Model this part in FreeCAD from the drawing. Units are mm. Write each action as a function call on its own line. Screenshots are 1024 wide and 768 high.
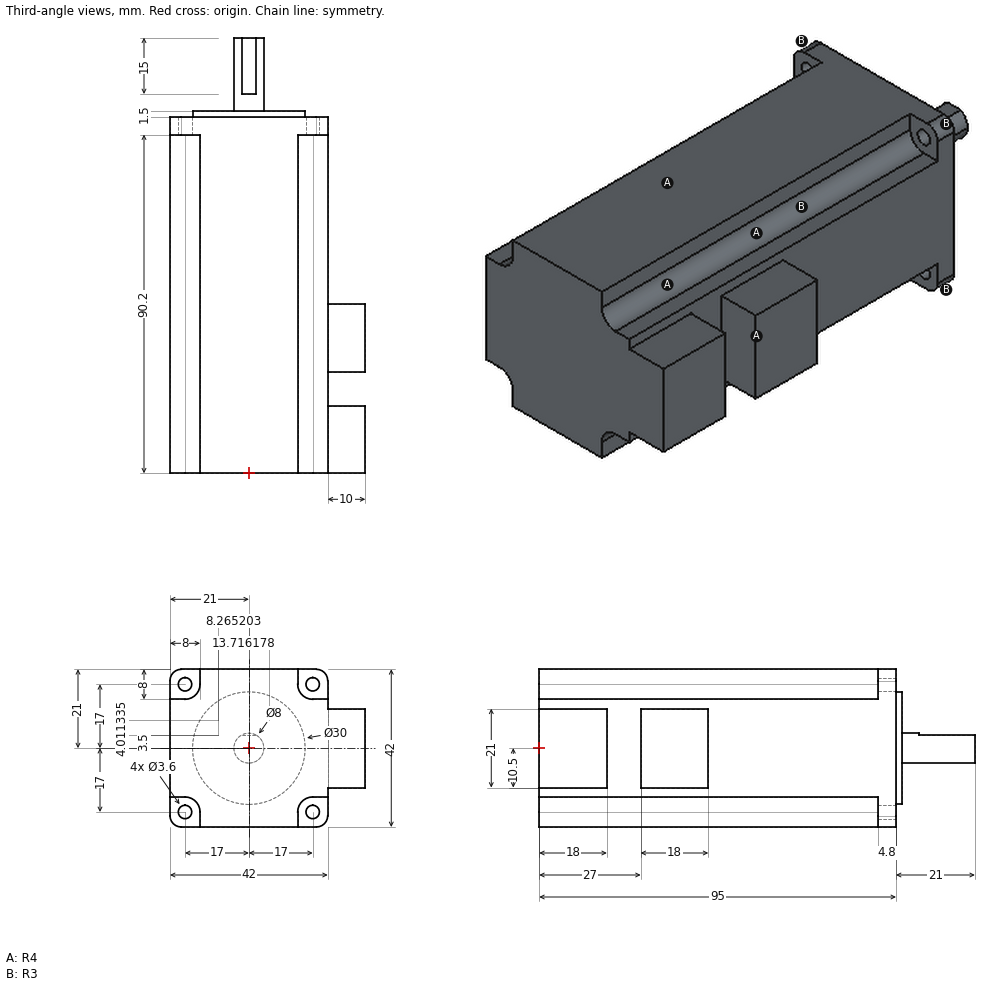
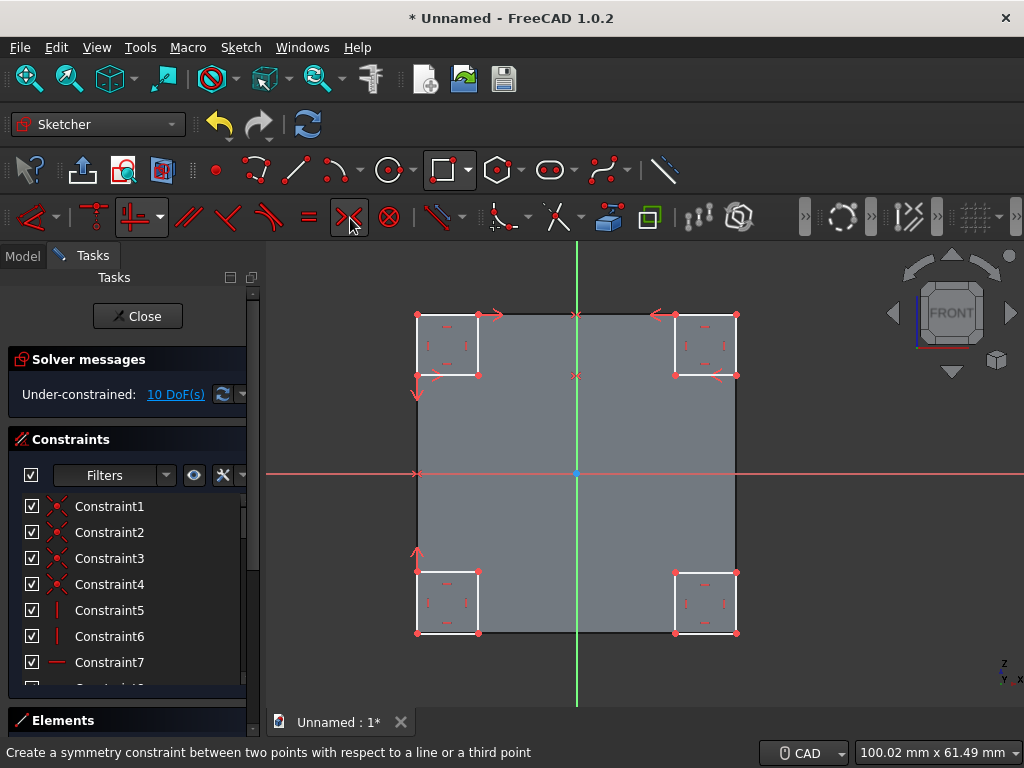
click(478, 315)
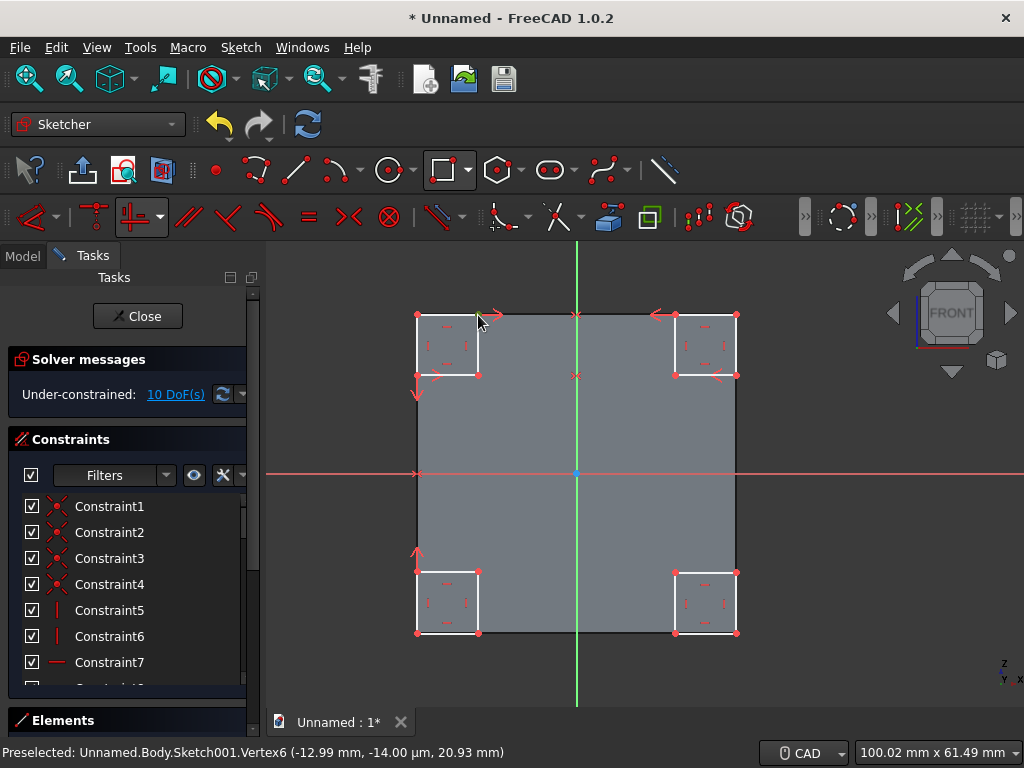
click(478, 634)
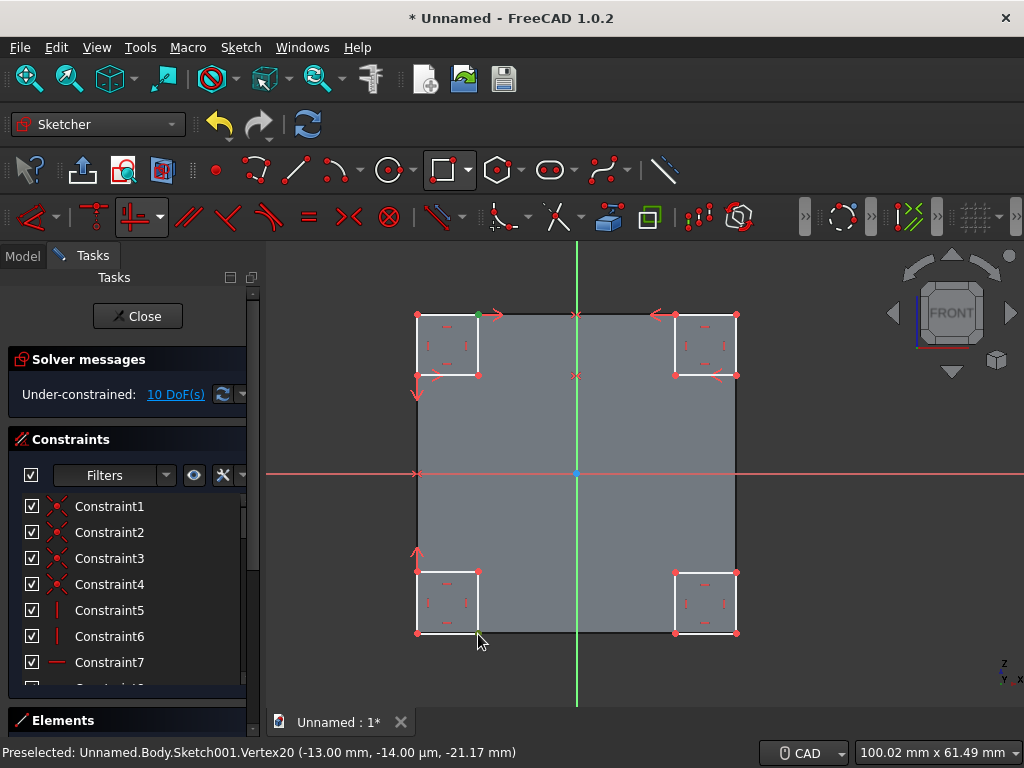
click(334, 474)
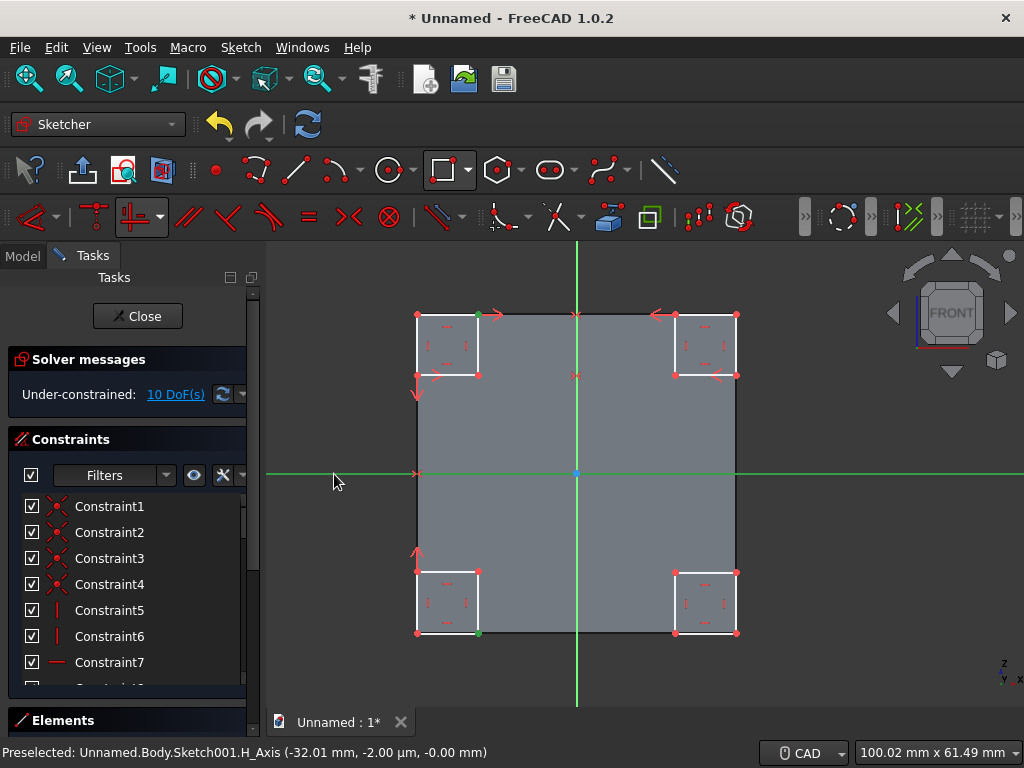
click(350, 218)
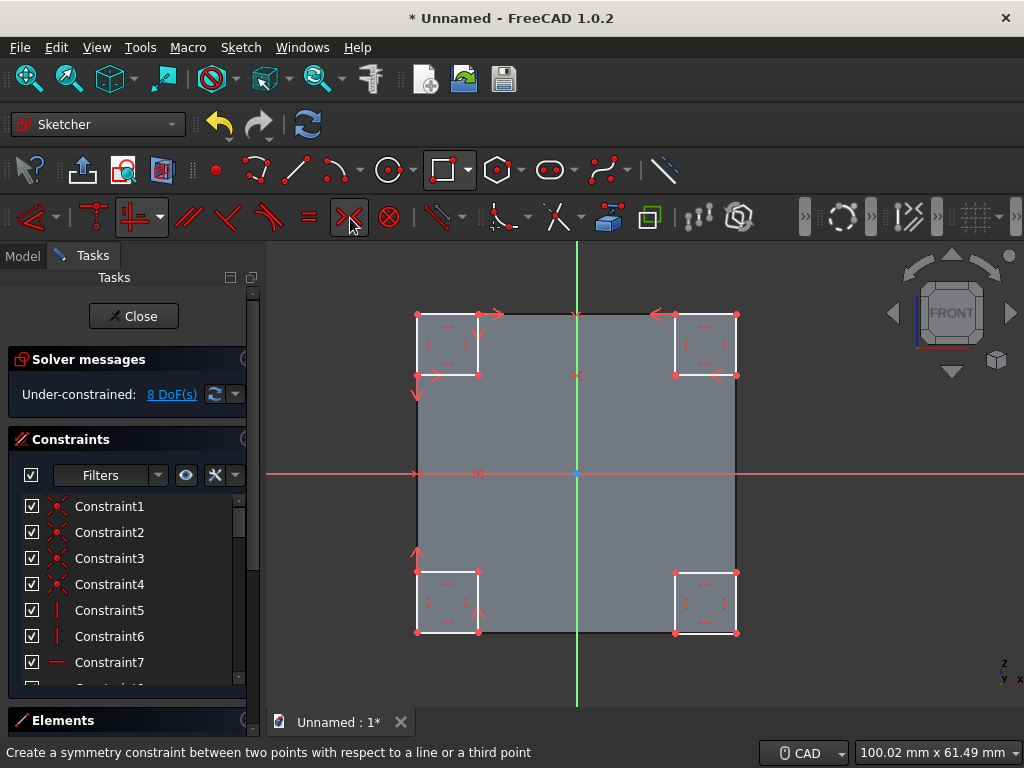
click(675, 375)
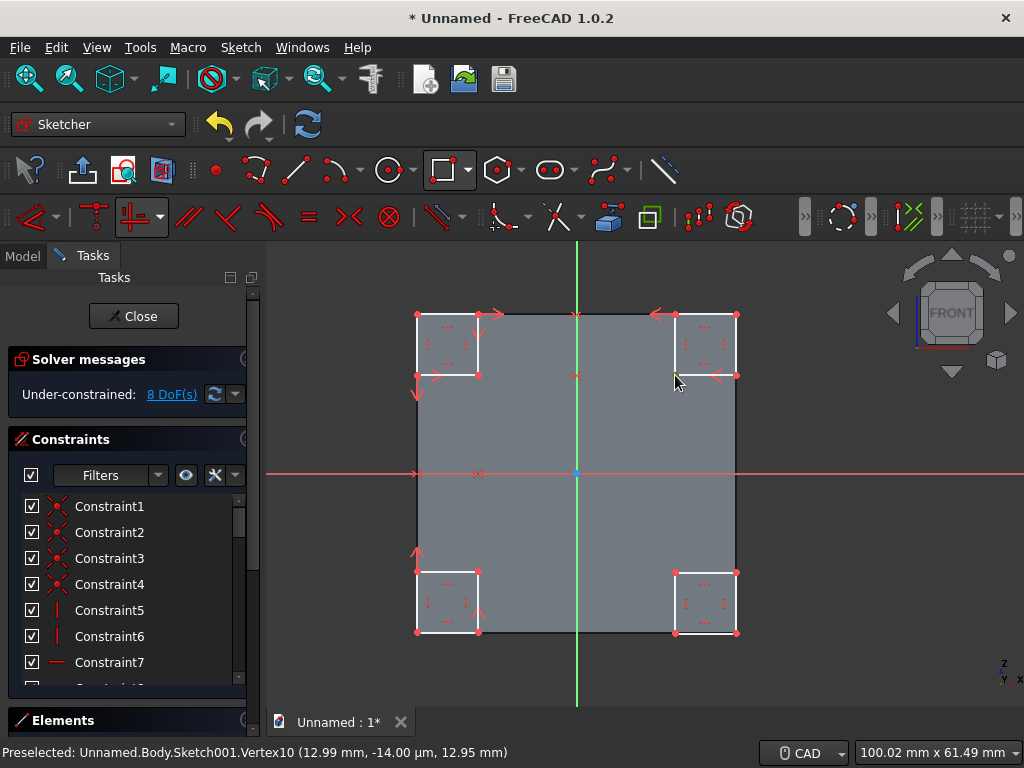
click(675, 573)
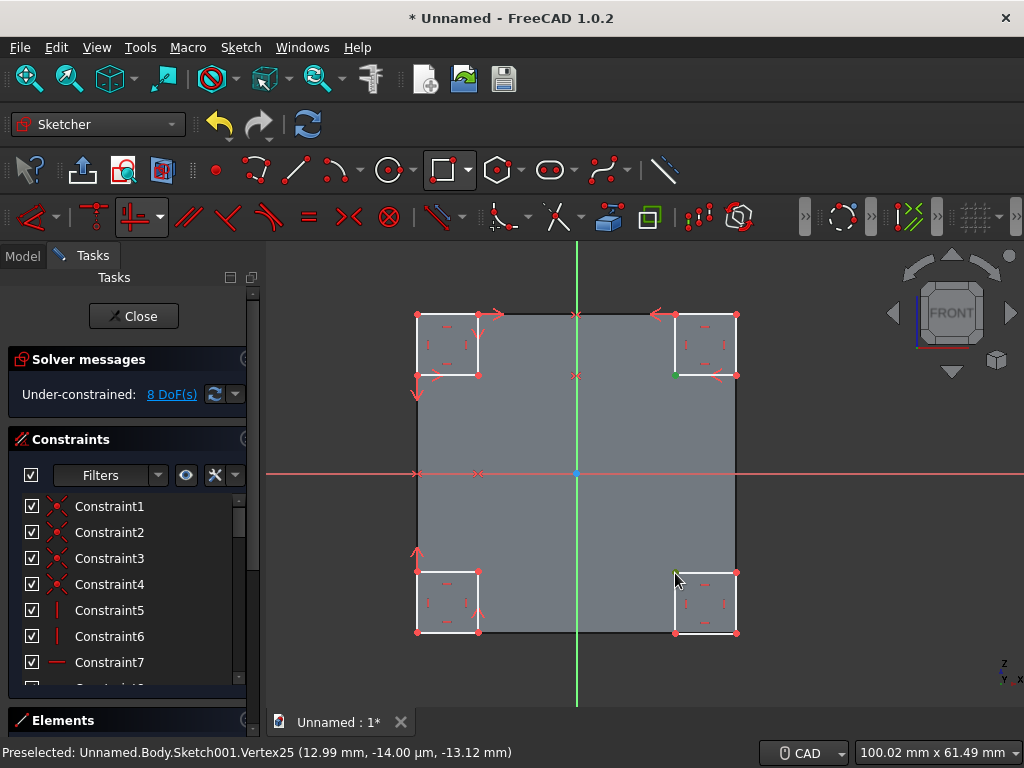
click(334, 474)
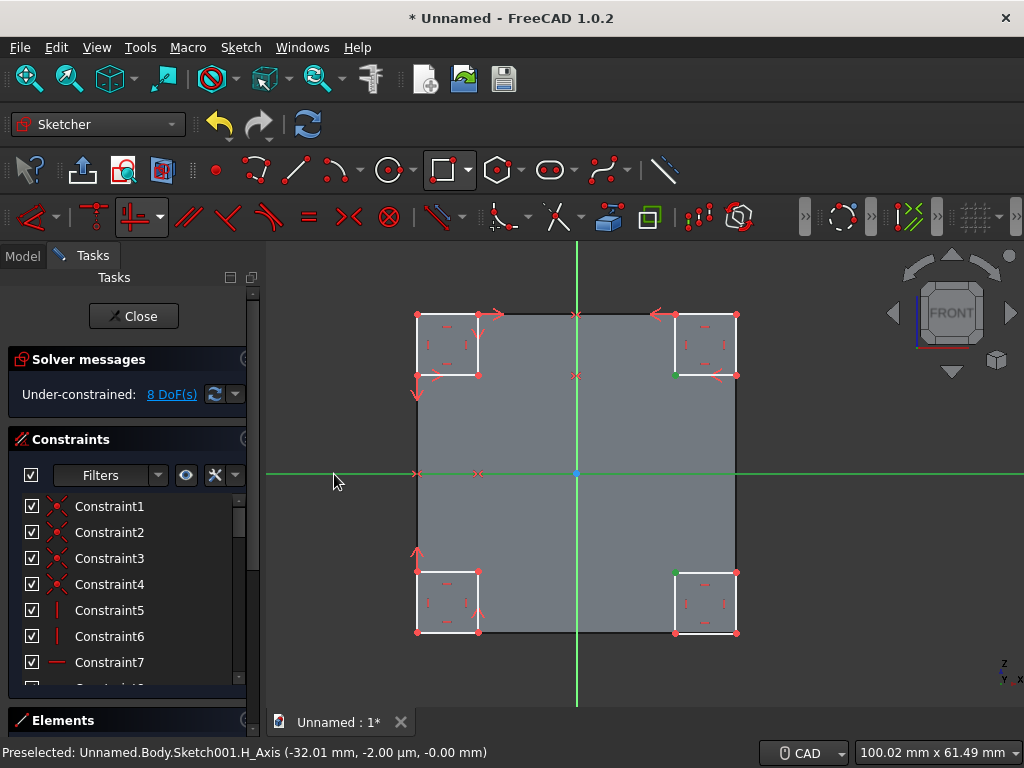
click(350, 218)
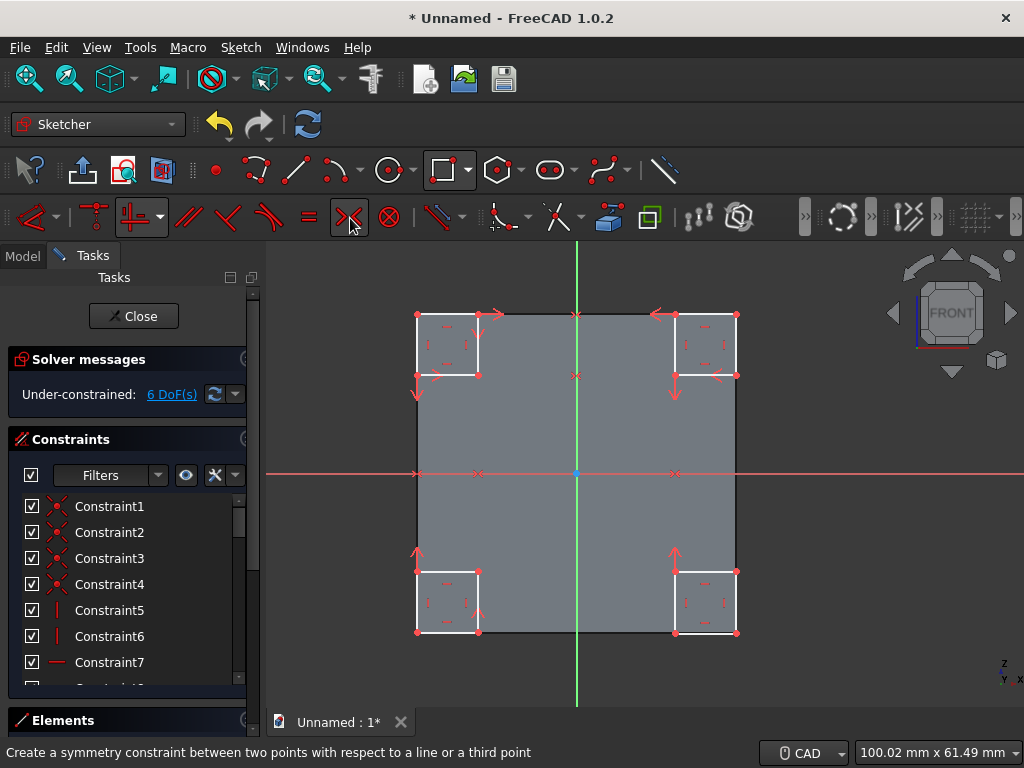
click(736, 314)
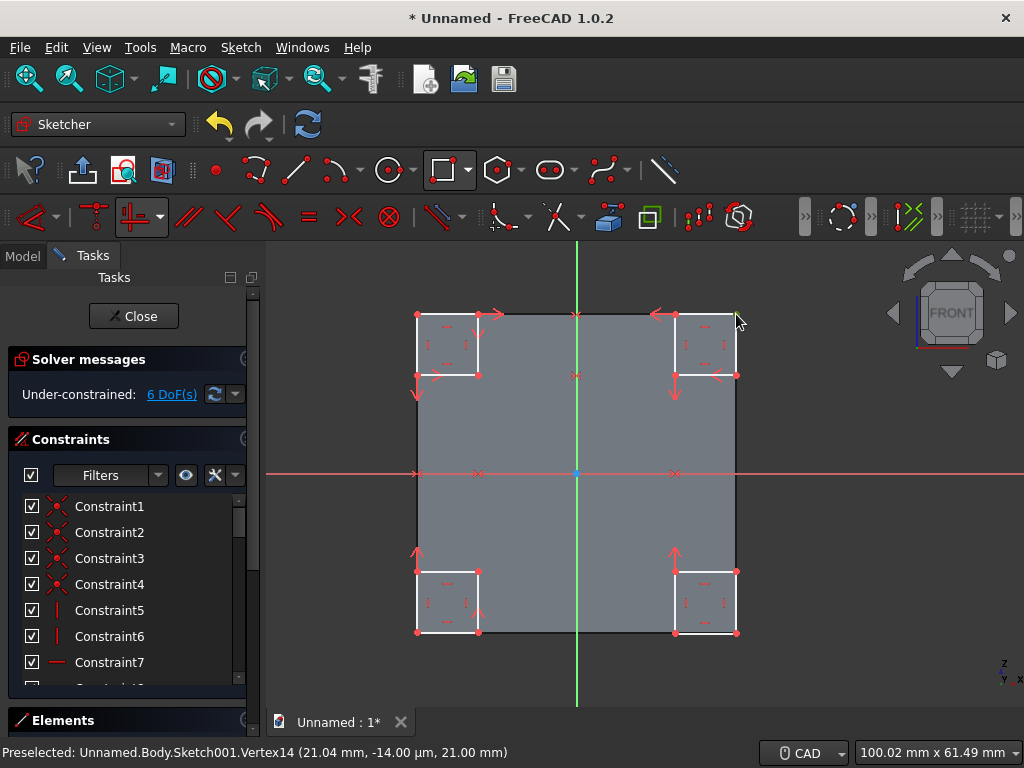
click(736, 634)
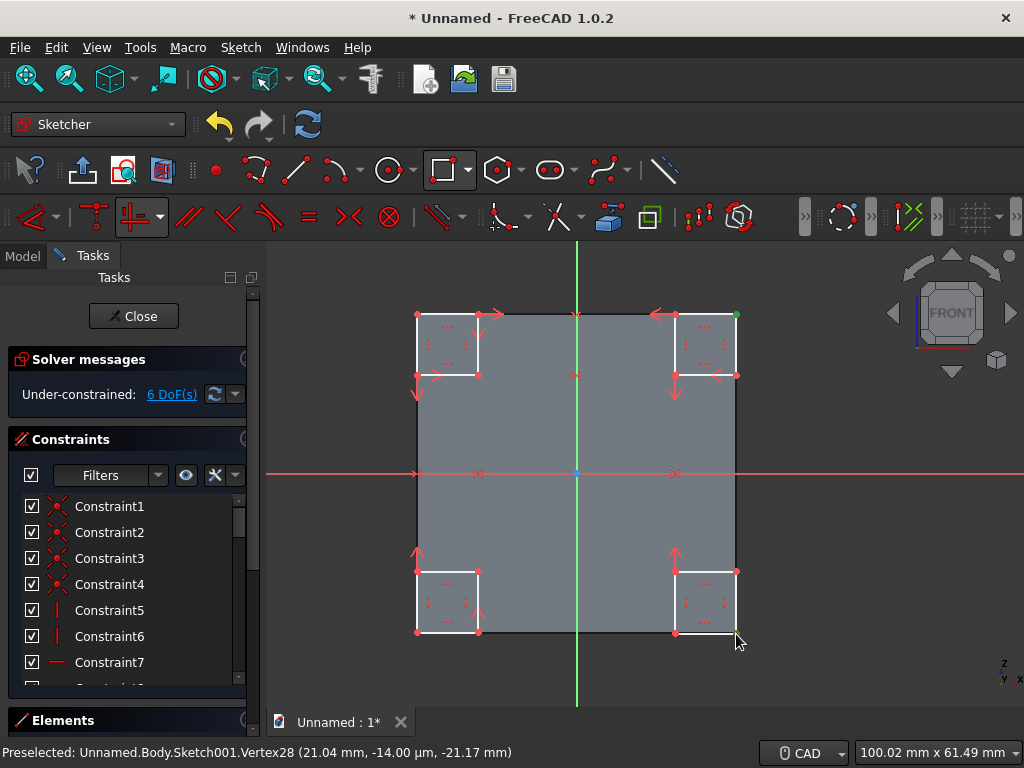
click(334, 474)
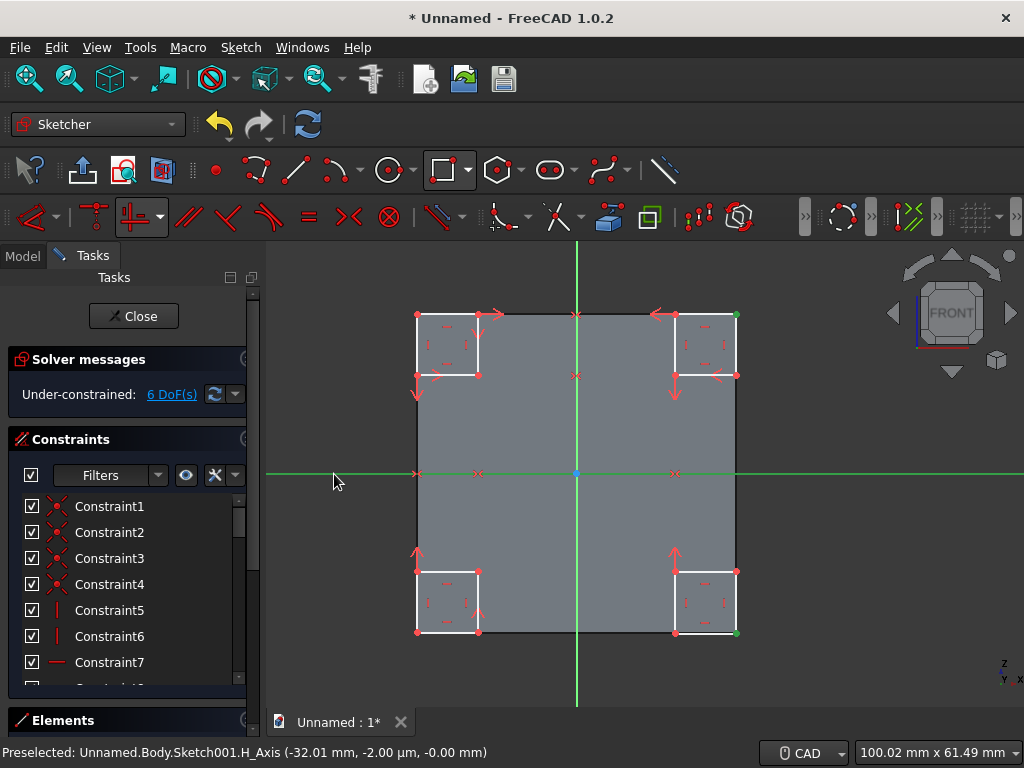
click(350, 218)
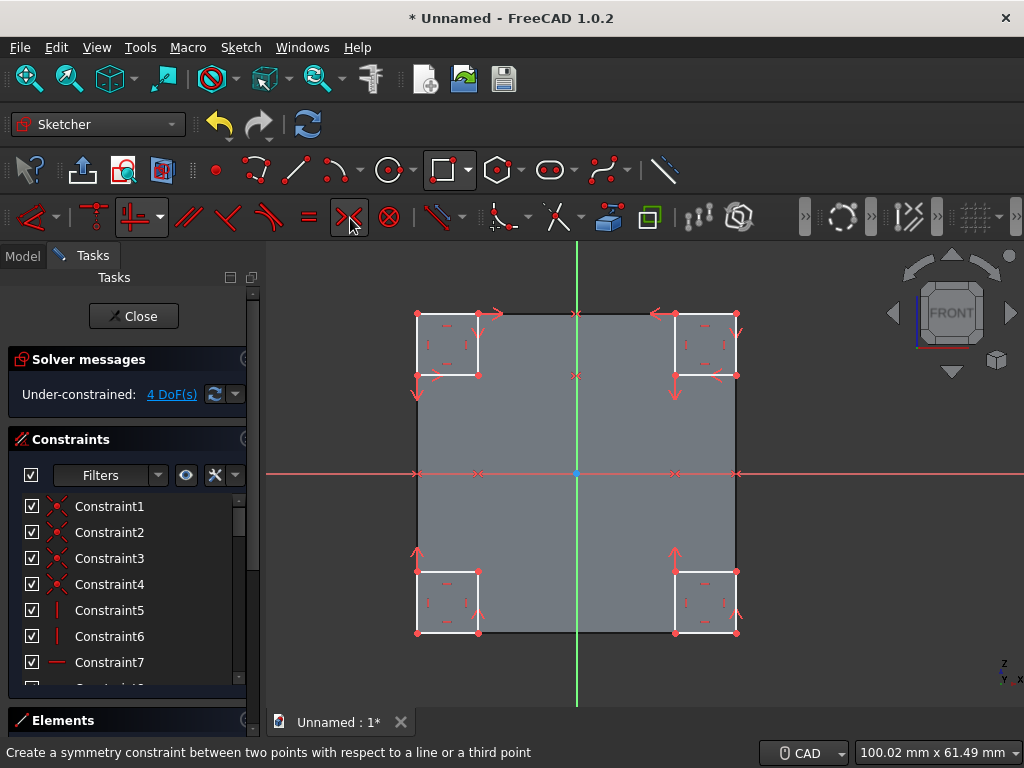
click(32, 218)